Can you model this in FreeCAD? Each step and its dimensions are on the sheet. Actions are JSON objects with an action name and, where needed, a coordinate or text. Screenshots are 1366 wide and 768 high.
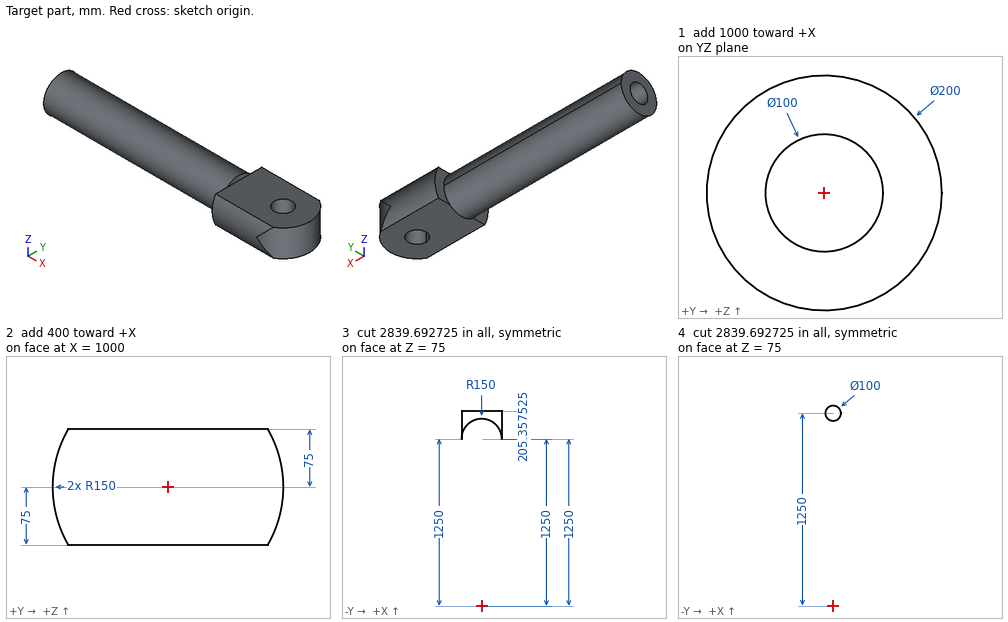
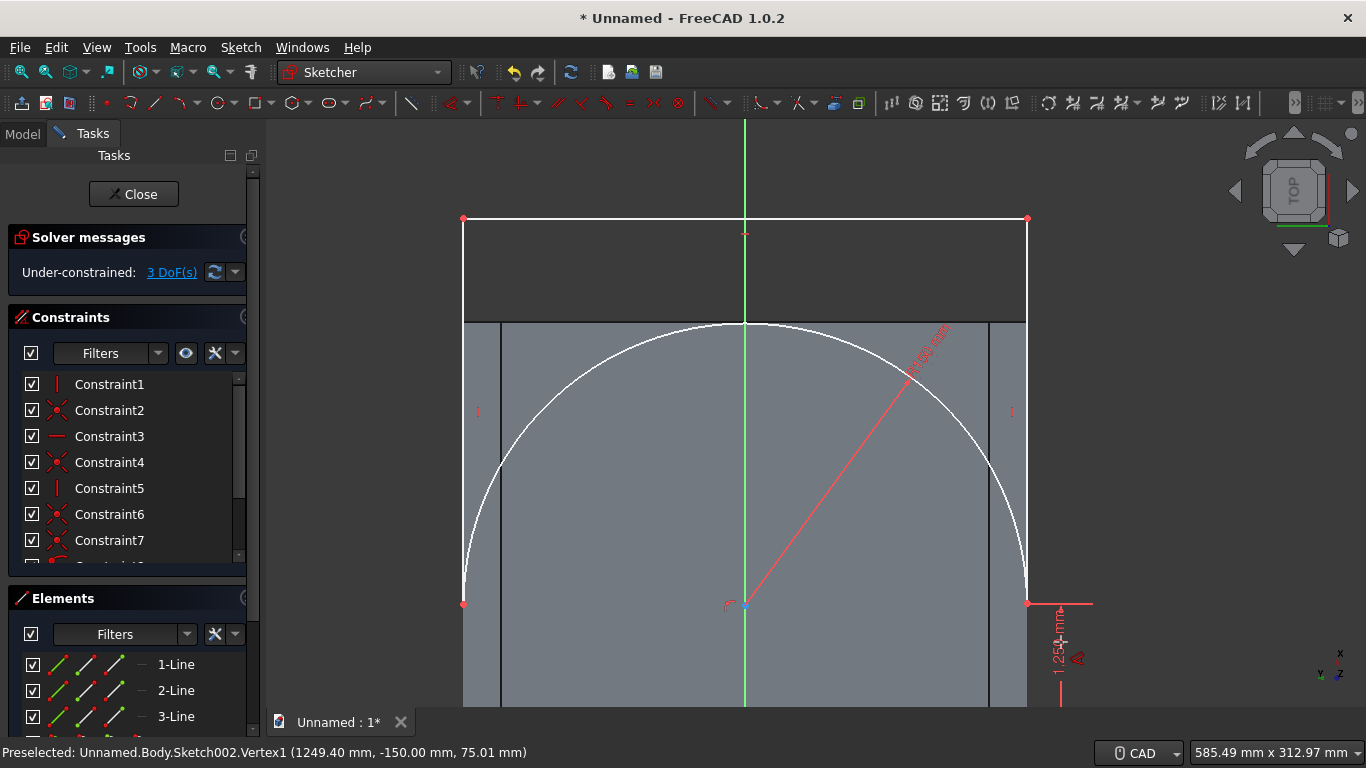
{"action": "left_click", "coordinate": [463, 605]}
{"action": "left_click", "coordinate": [429, 642]}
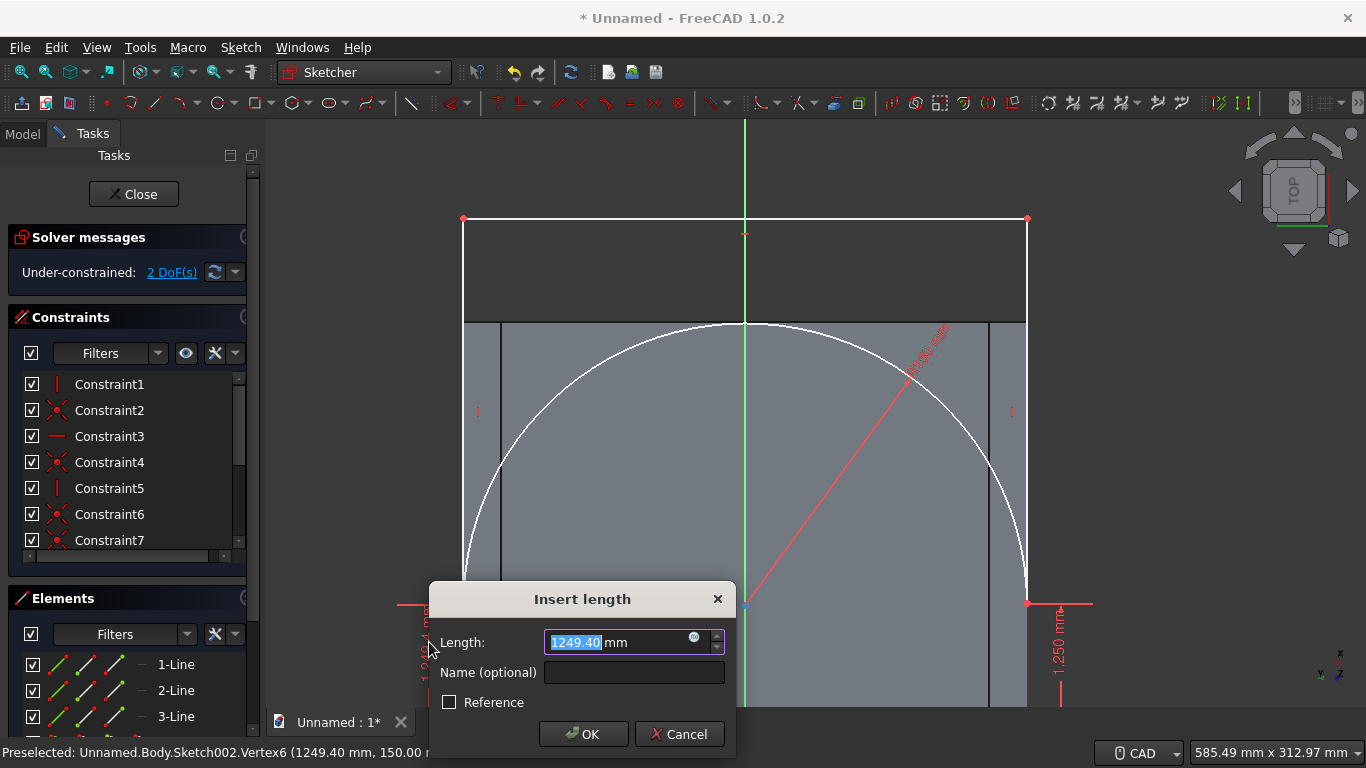
{"action": "type", "text": "1250"}
{"action": "key", "text": "Return"}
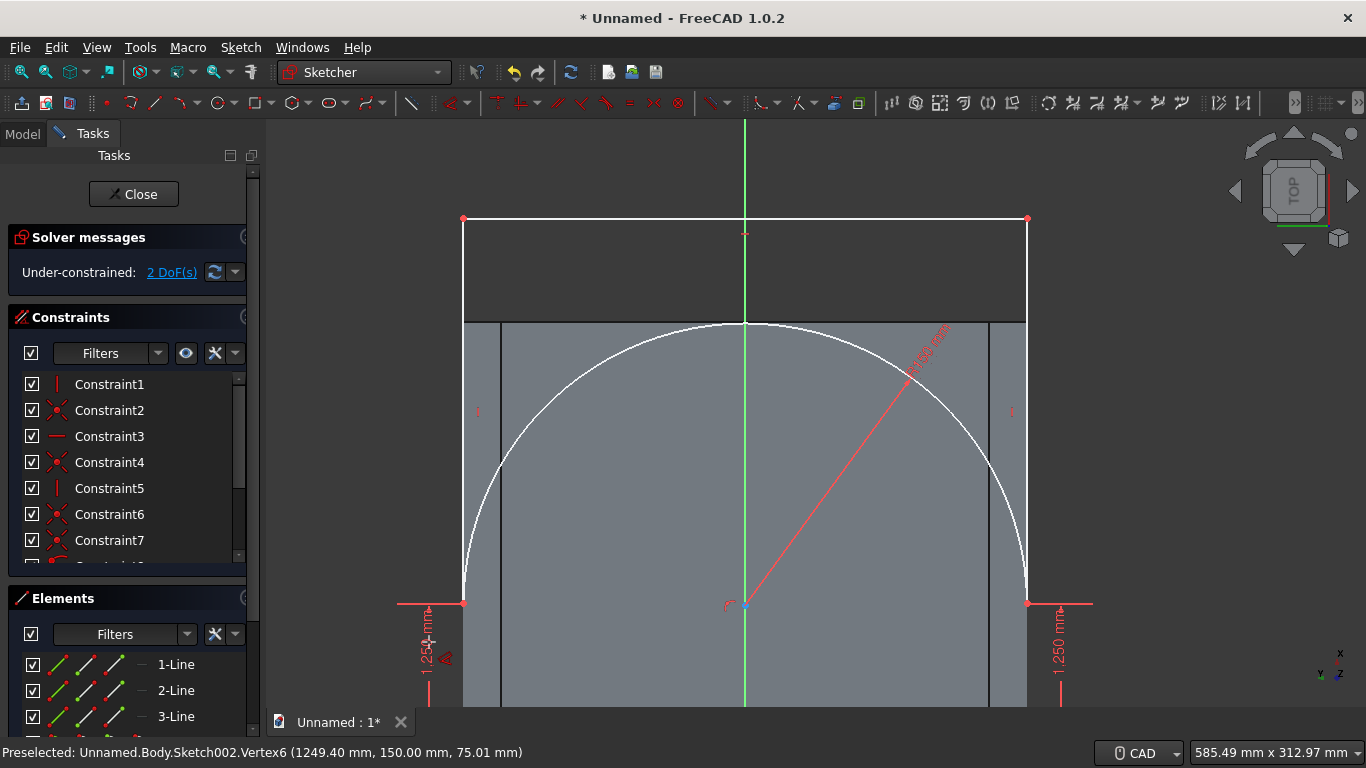
{"action": "left_click", "coordinate": [745, 605]}
{"action": "left_click", "coordinate": [779, 642]}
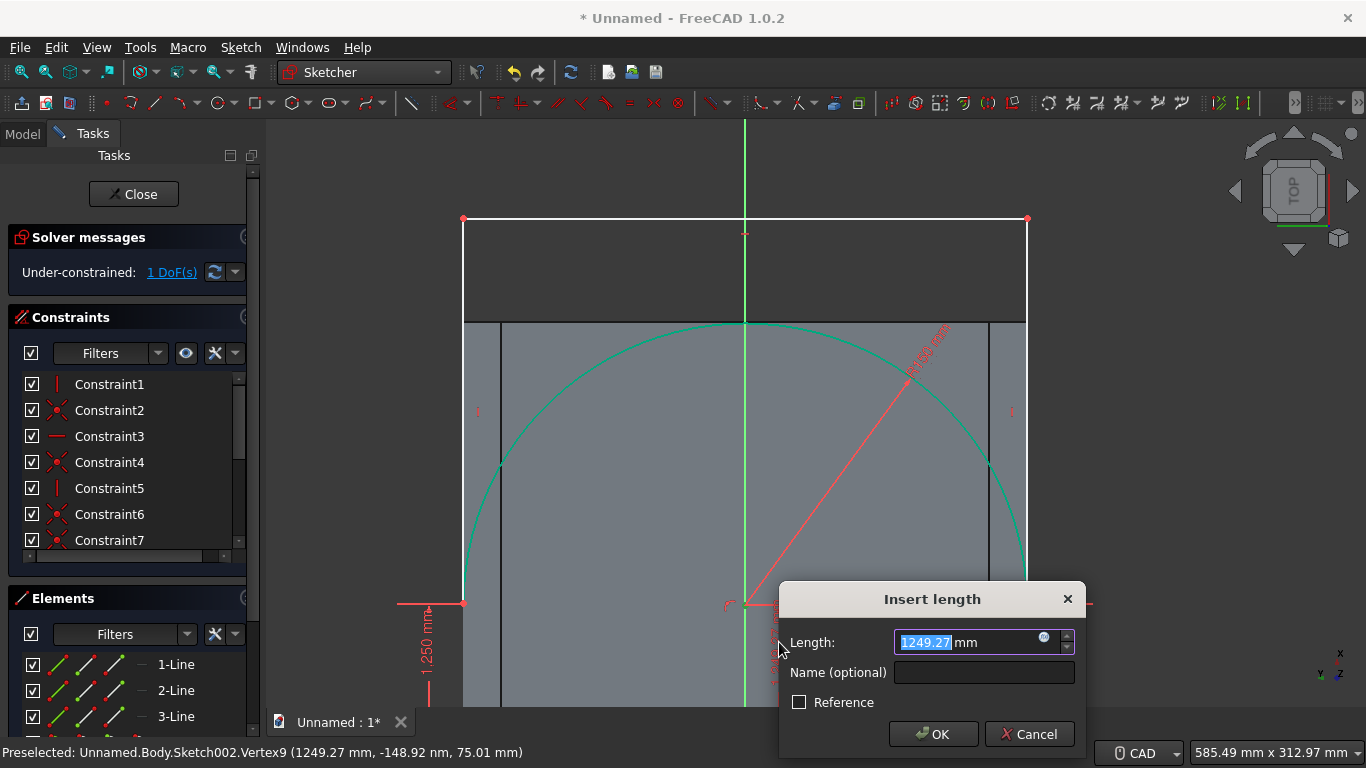
{"action": "type", "text": "1250"}
{"action": "key", "text": "Return"}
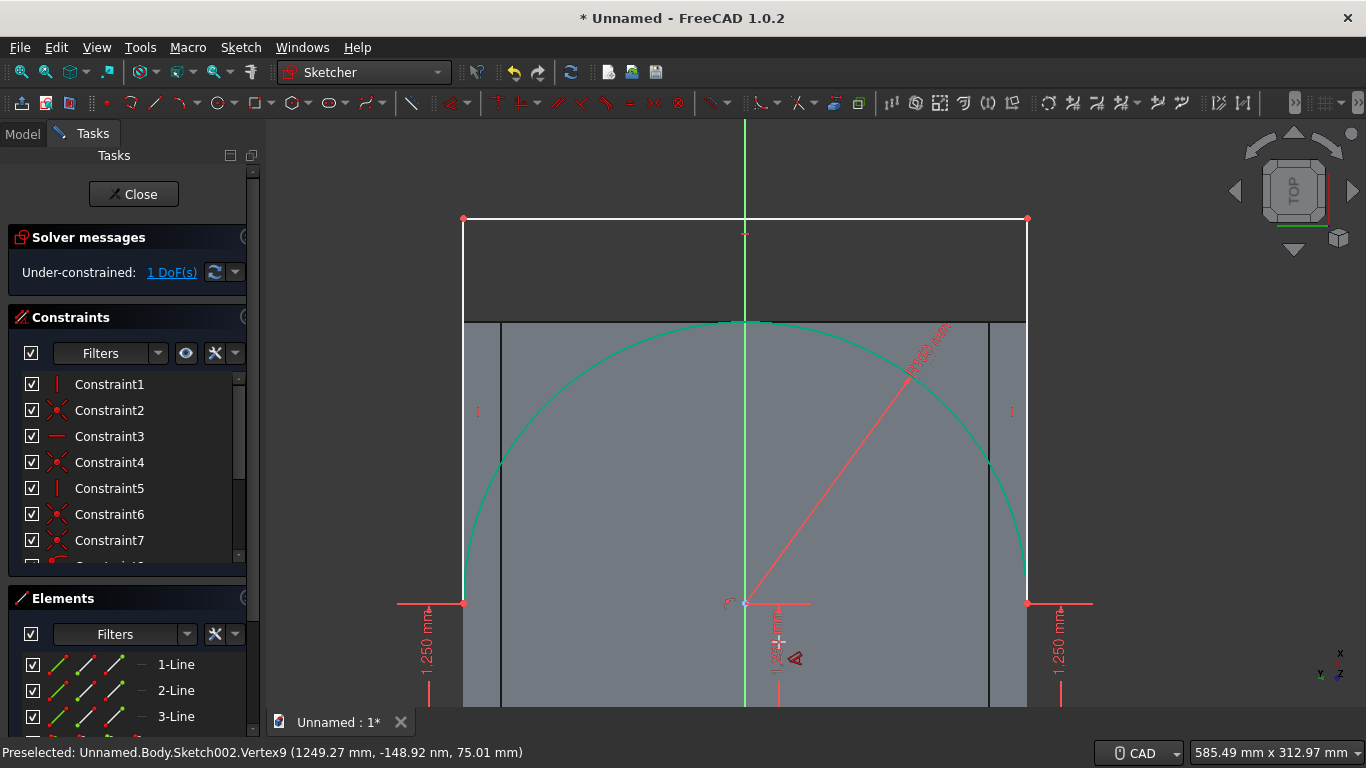
{"action": "left_click", "coordinate": [1027, 488]}
{"action": "left_click", "coordinate": [1061, 411]}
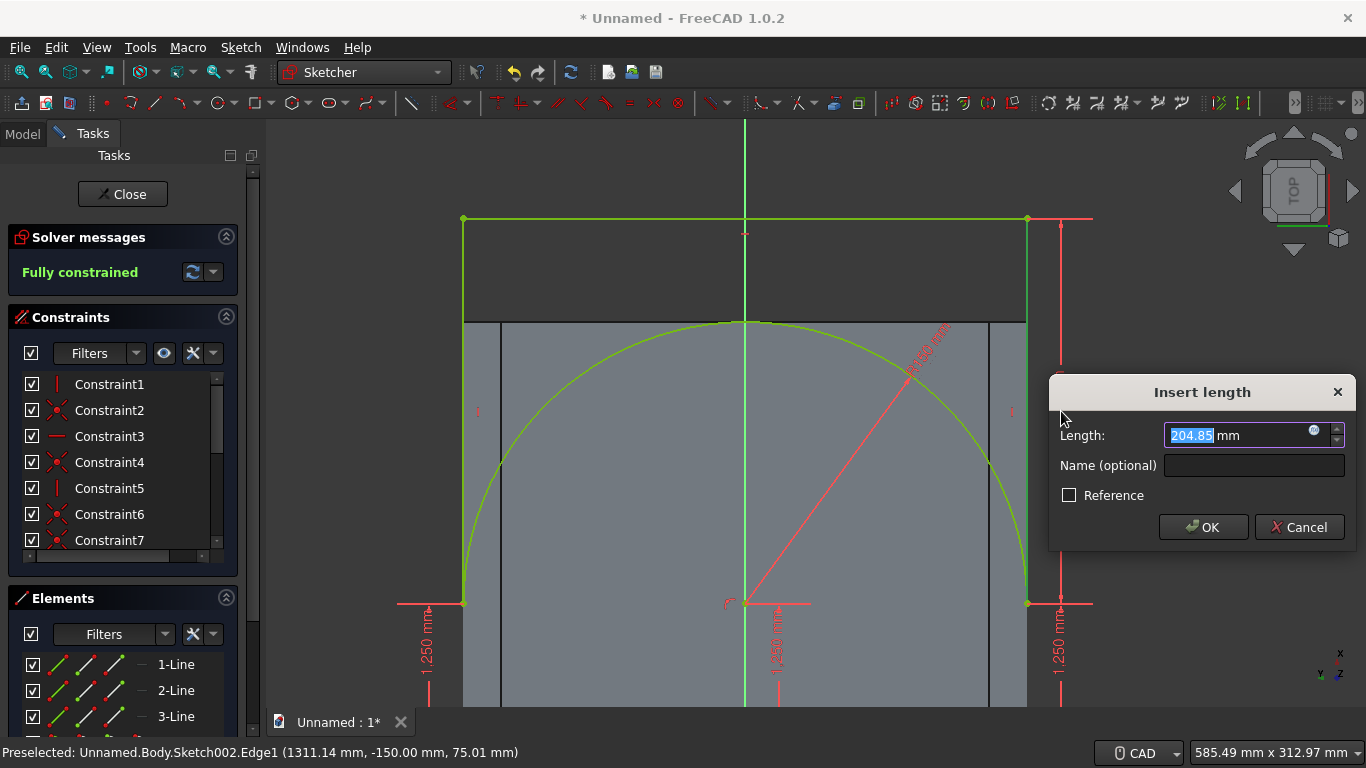
{"action": "type", "text": "205.357525"}
{"action": "key", "text": "Return"}
{"action": "key", "text": "Escape"}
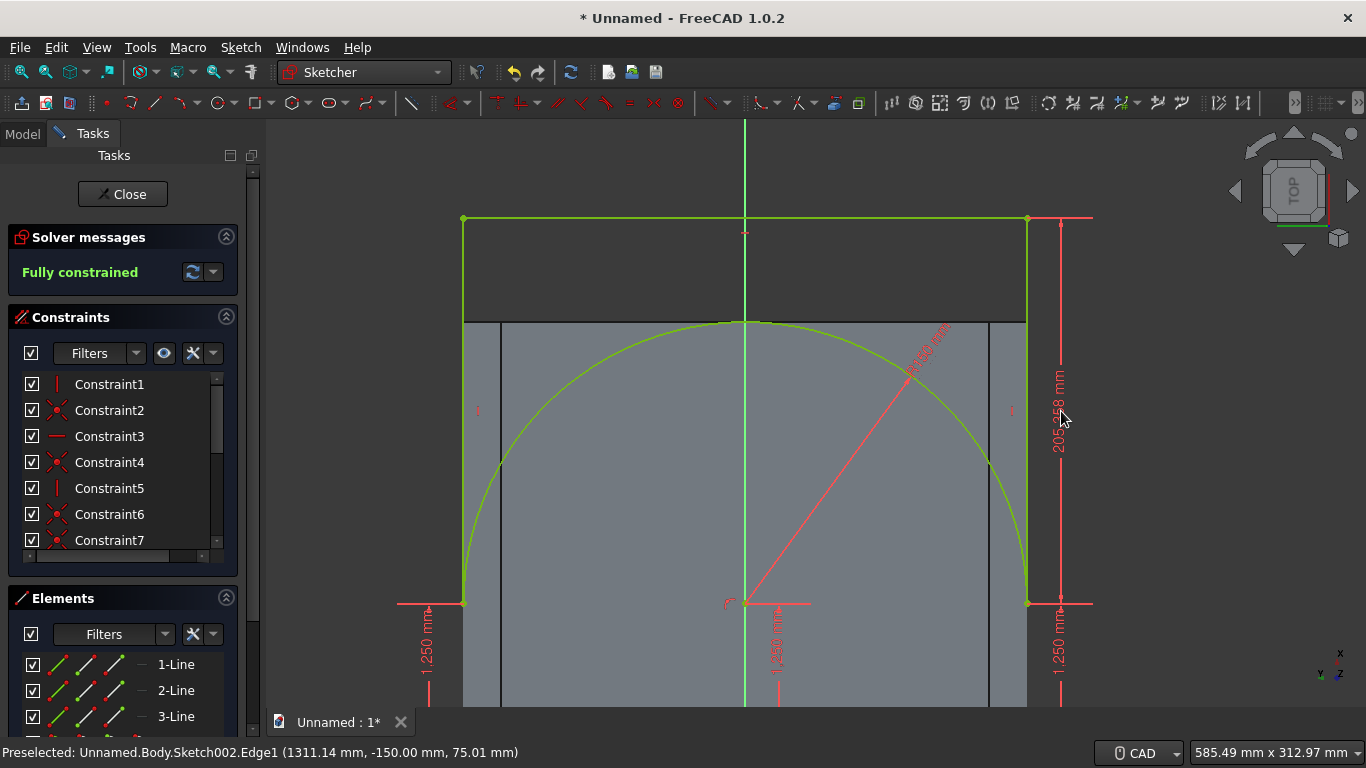
{"action": "left_click", "coordinate": [123, 194]}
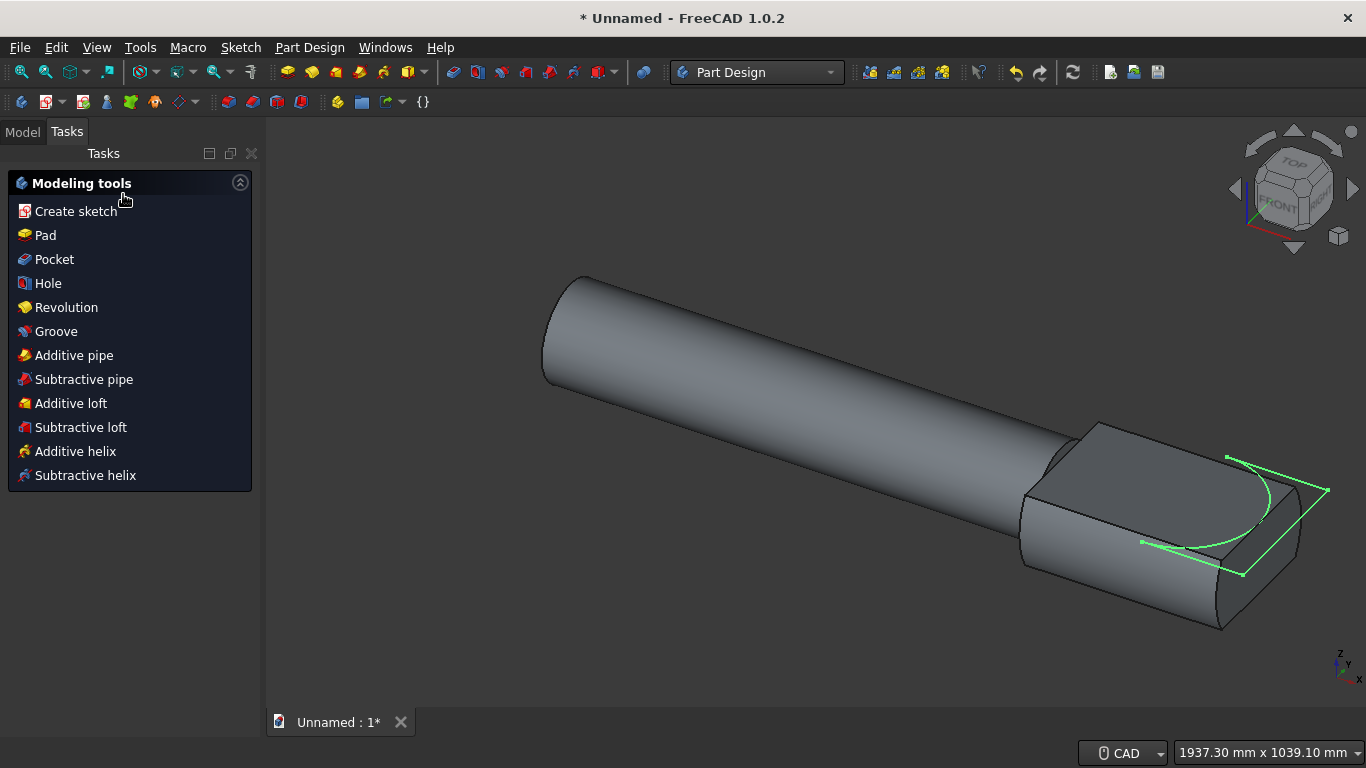
{"action": "left_click", "coordinate": [454, 72]}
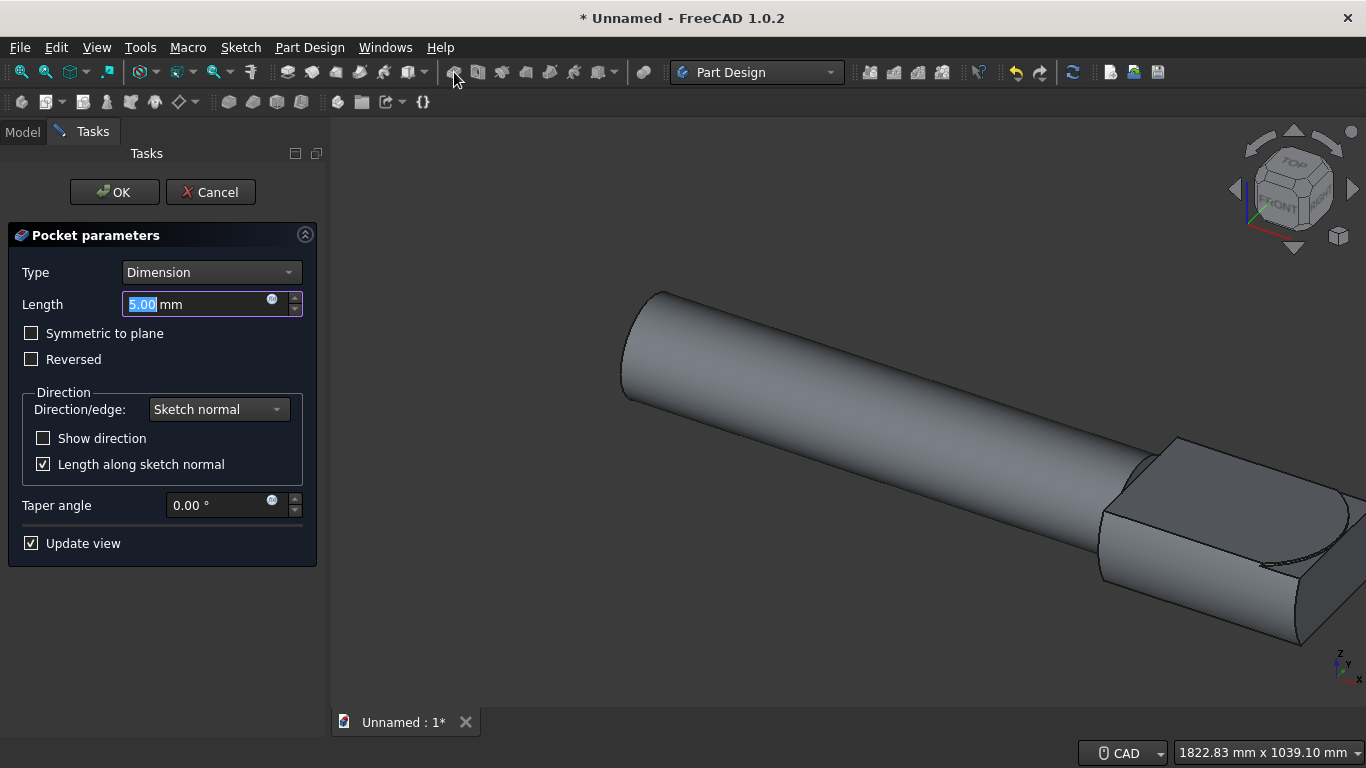
{"action": "type", "text": "2839.692725"}
{"action": "key", "text": "Tab"}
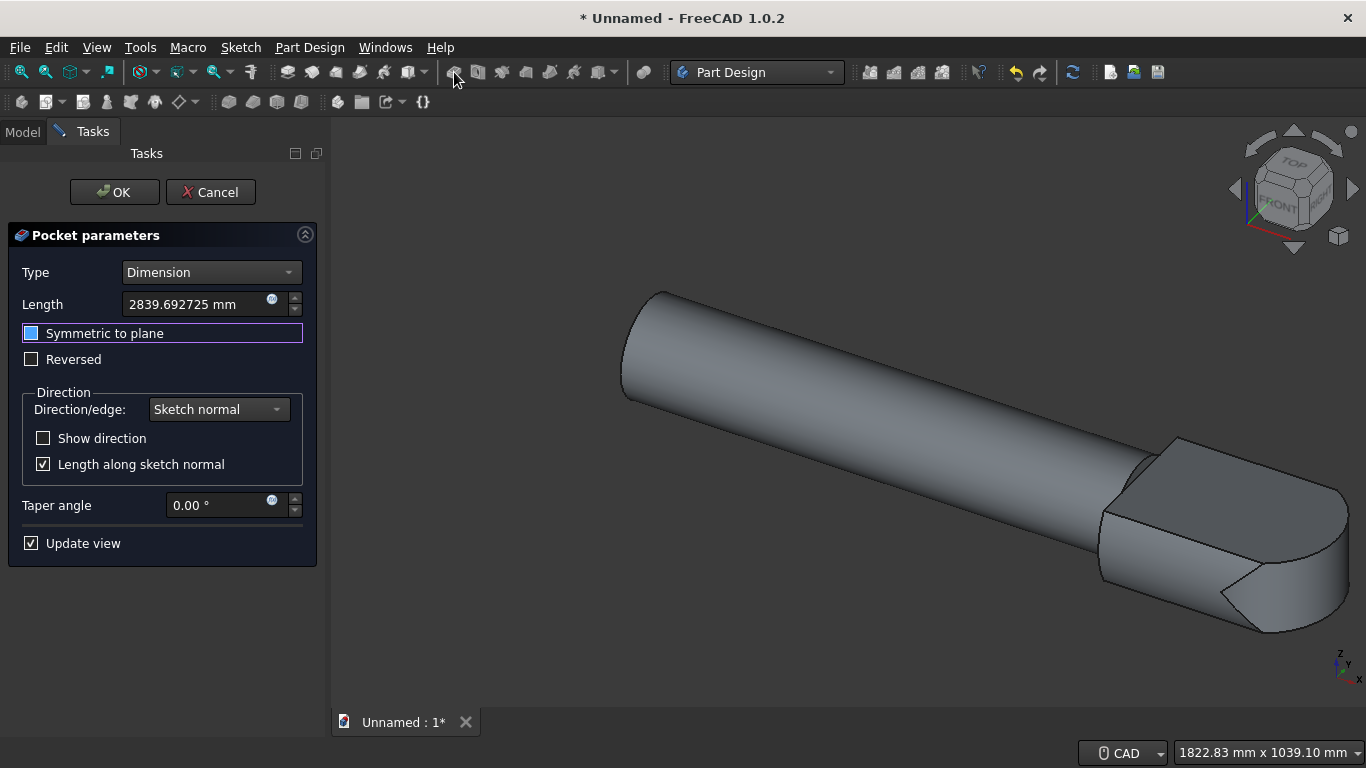
{"action": "left_click", "coordinate": [30, 333]}